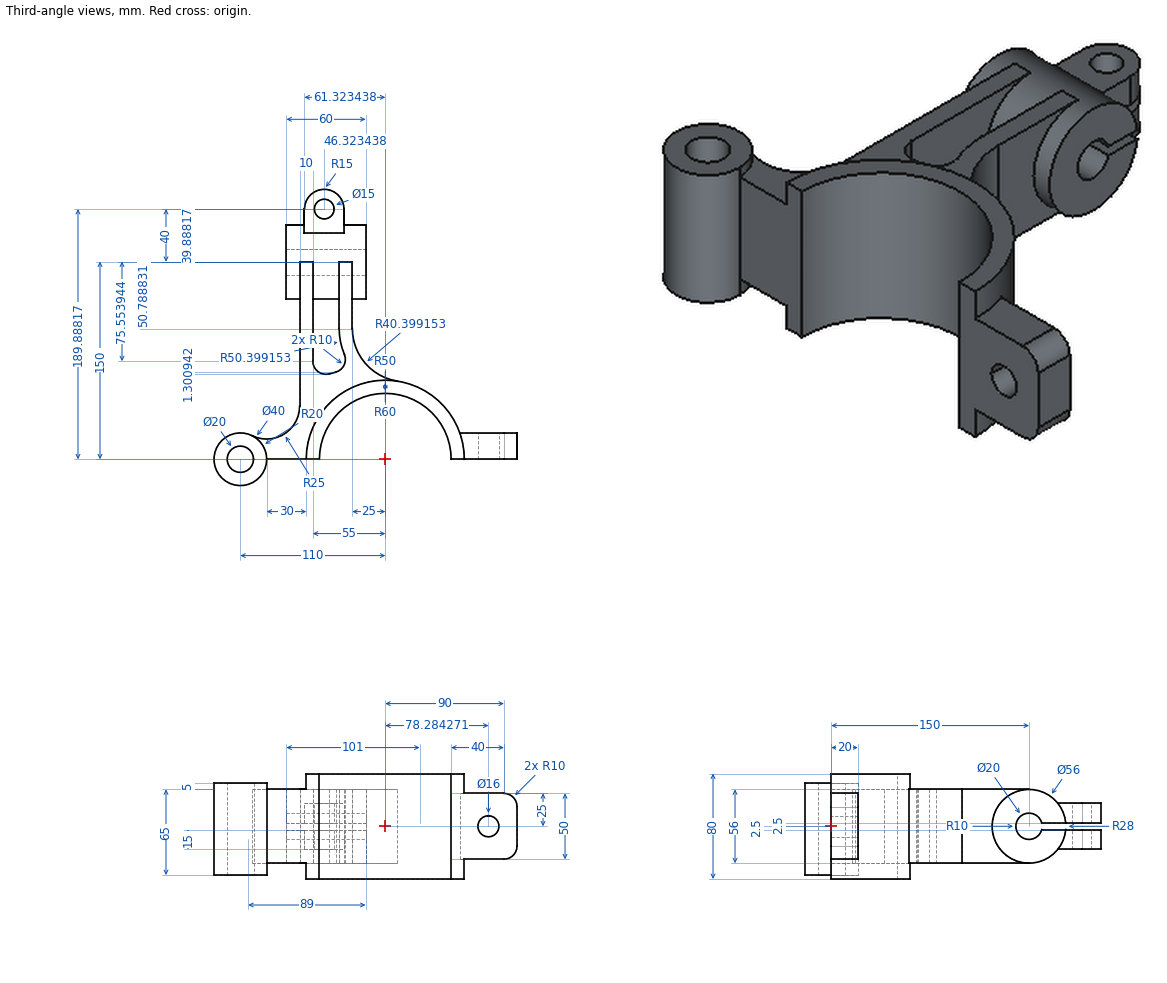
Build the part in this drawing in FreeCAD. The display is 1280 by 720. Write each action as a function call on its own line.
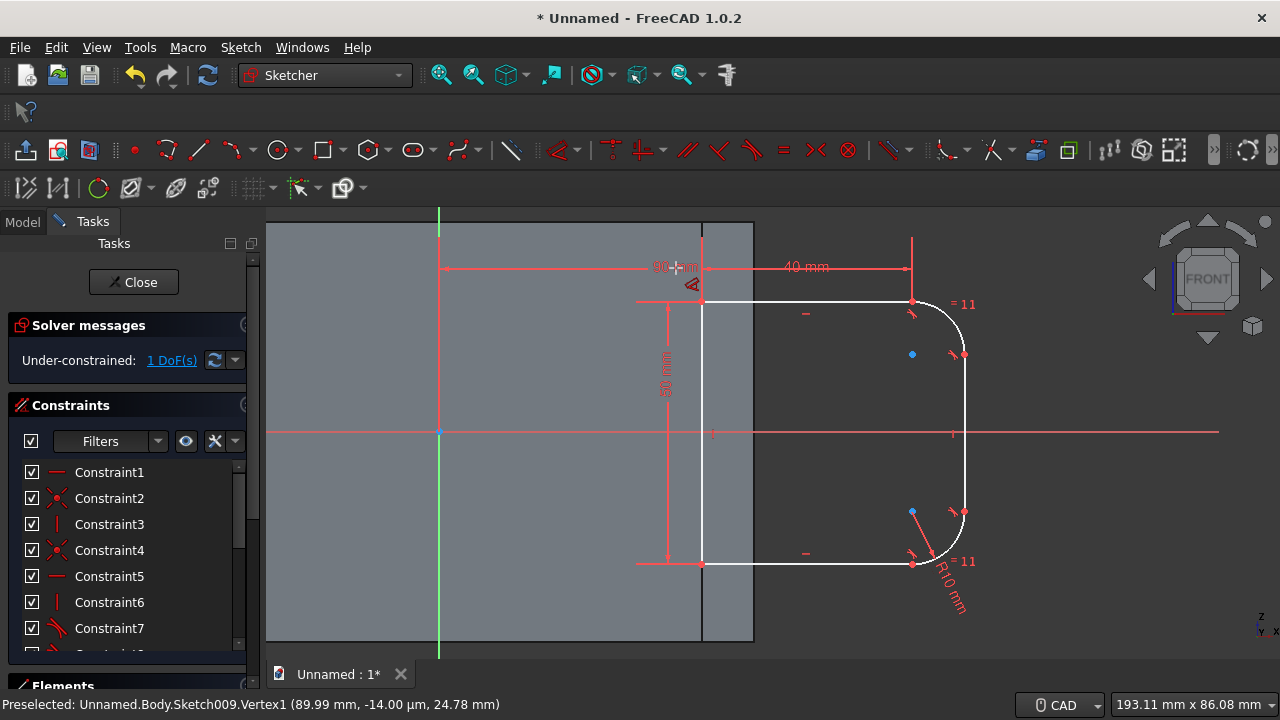
click(912, 302)
click(405, 367)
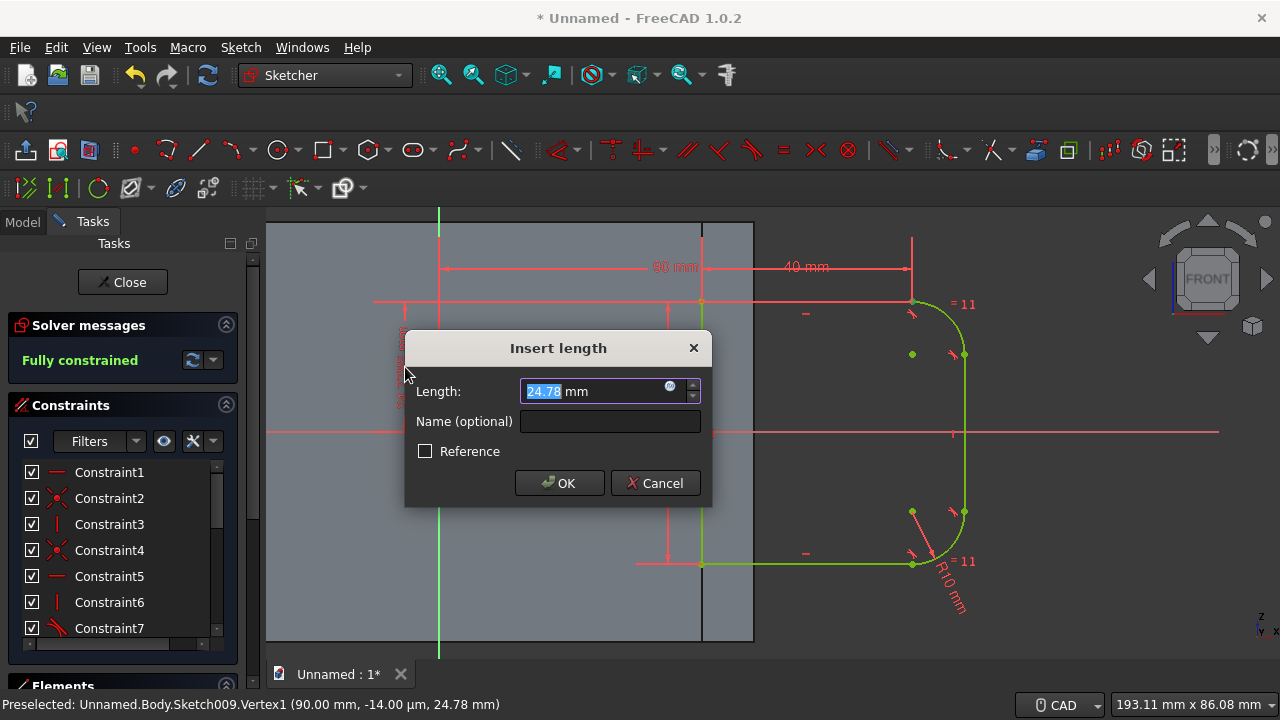
text(25)
key(Return)
key(Escape)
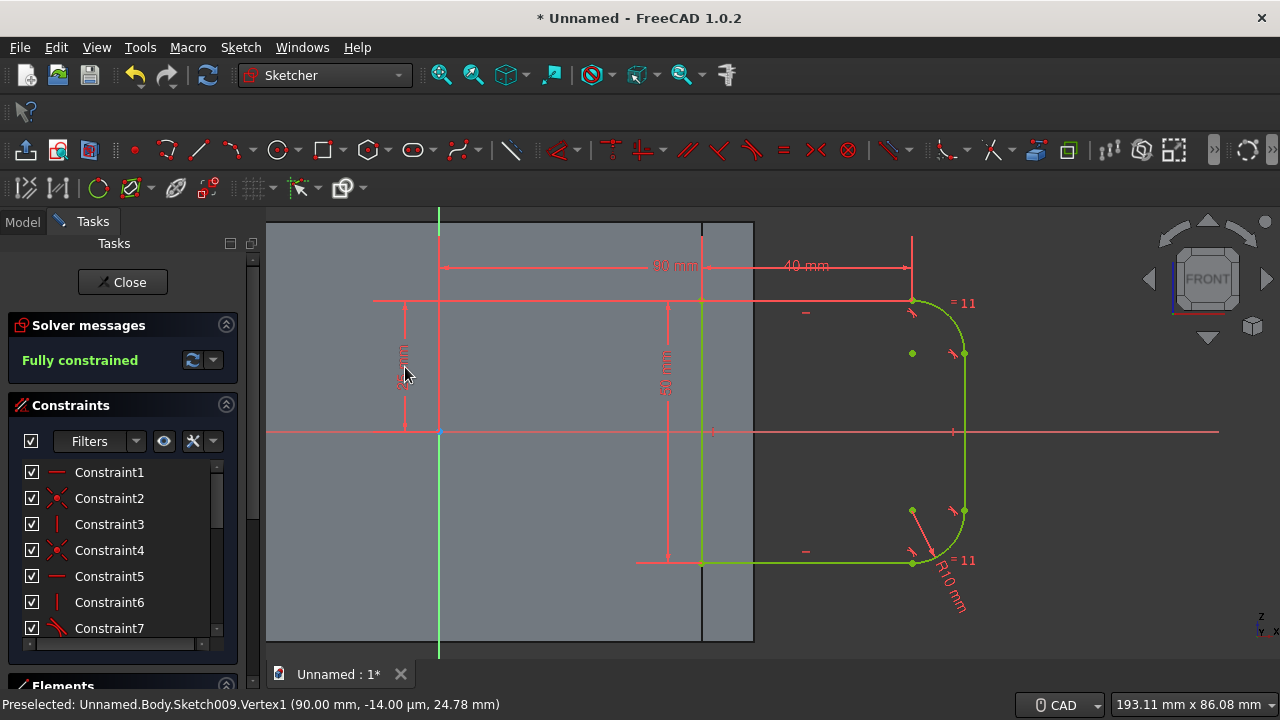
click(123, 282)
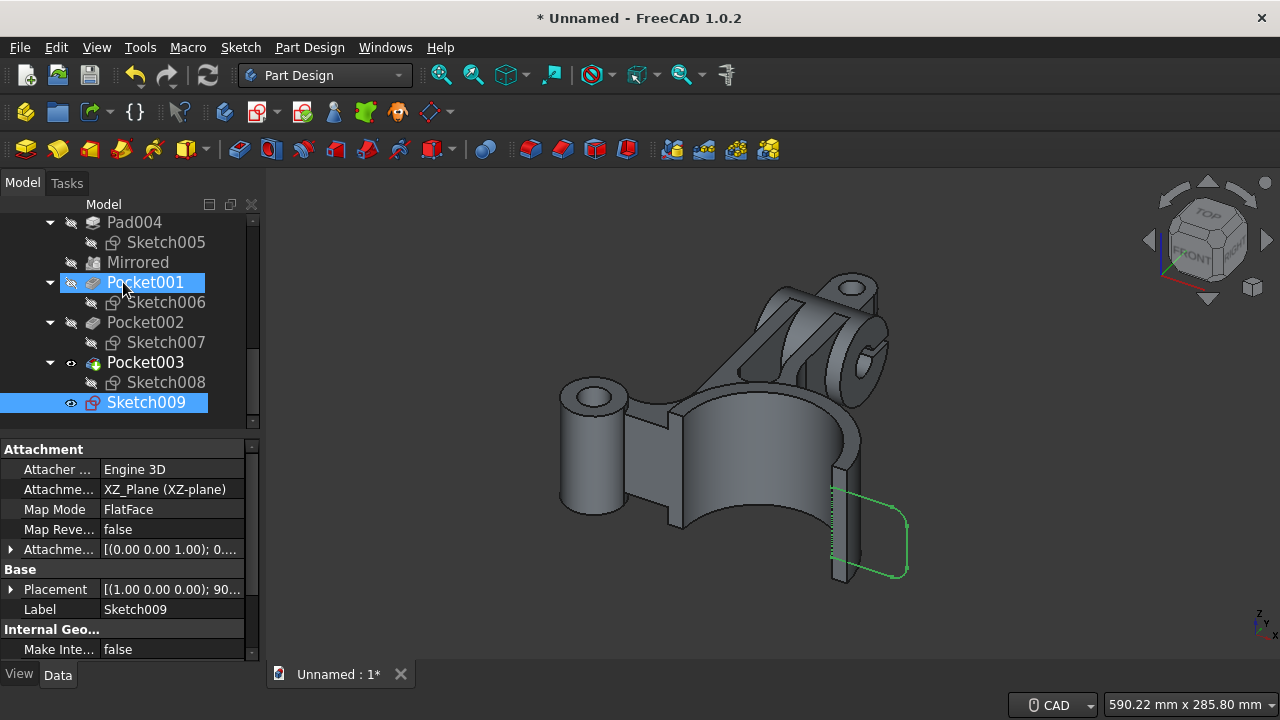
click(26, 150)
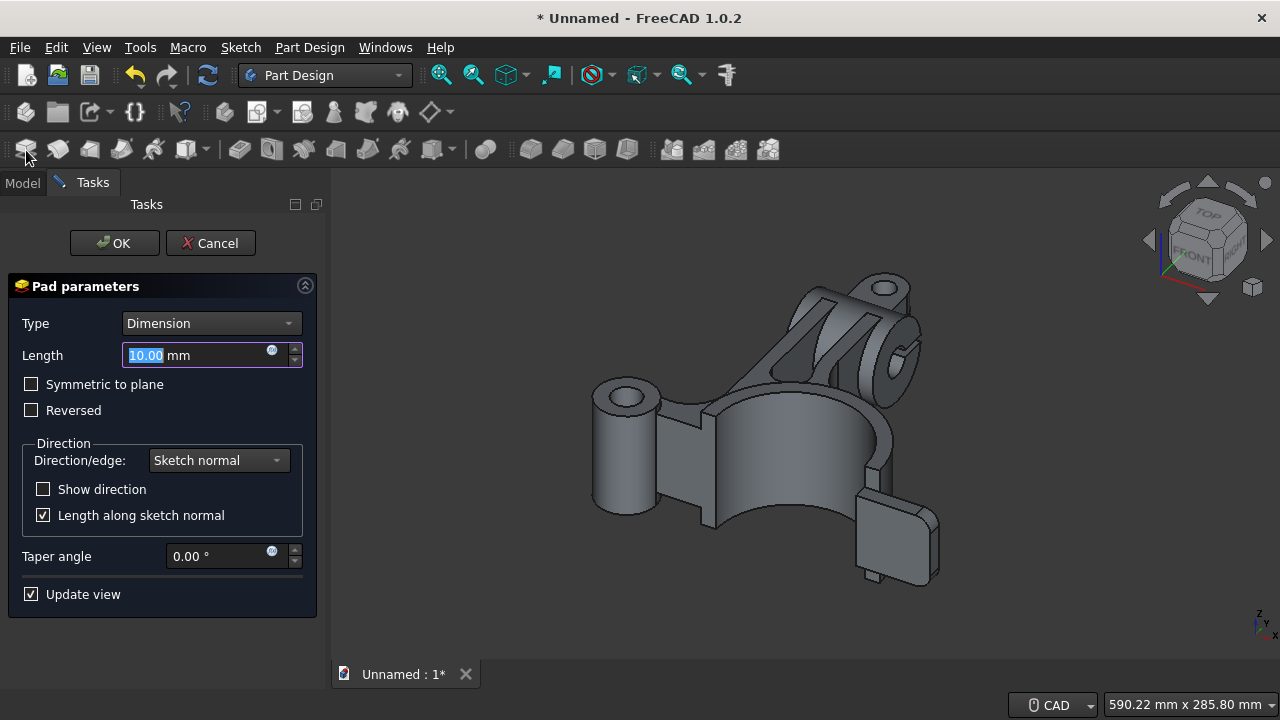
text(20)
key(Tab)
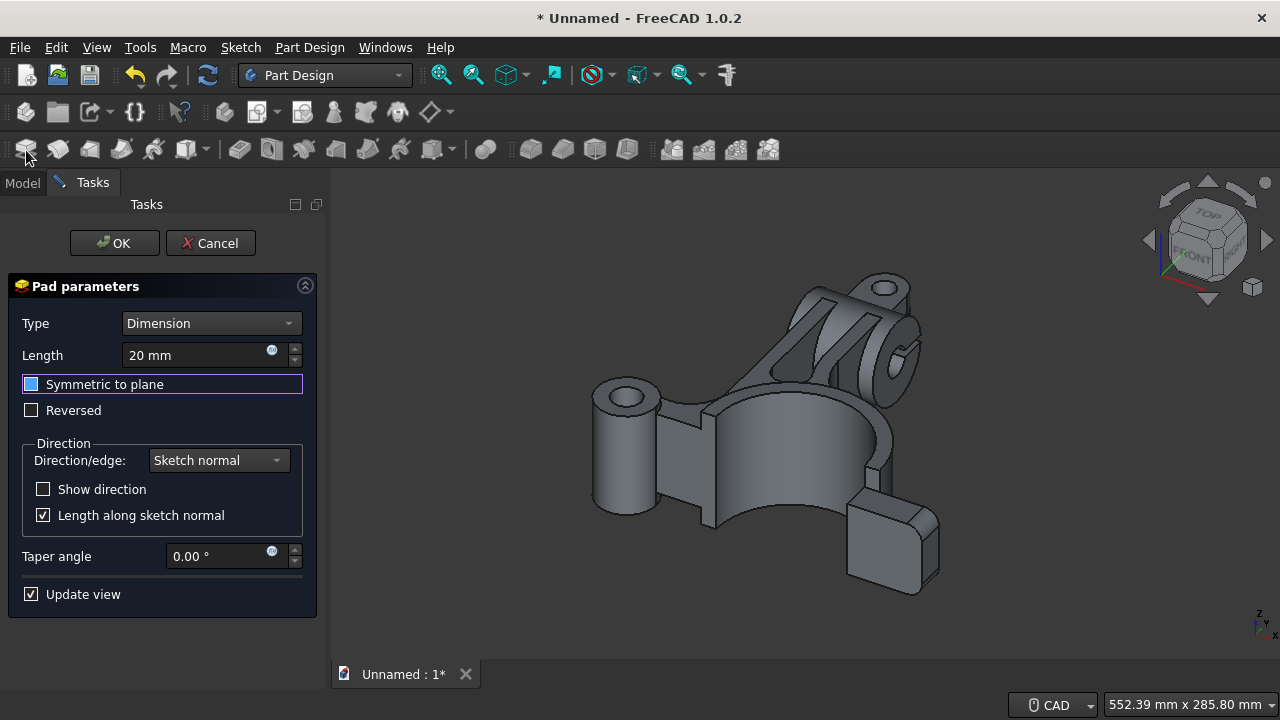
click(30, 410)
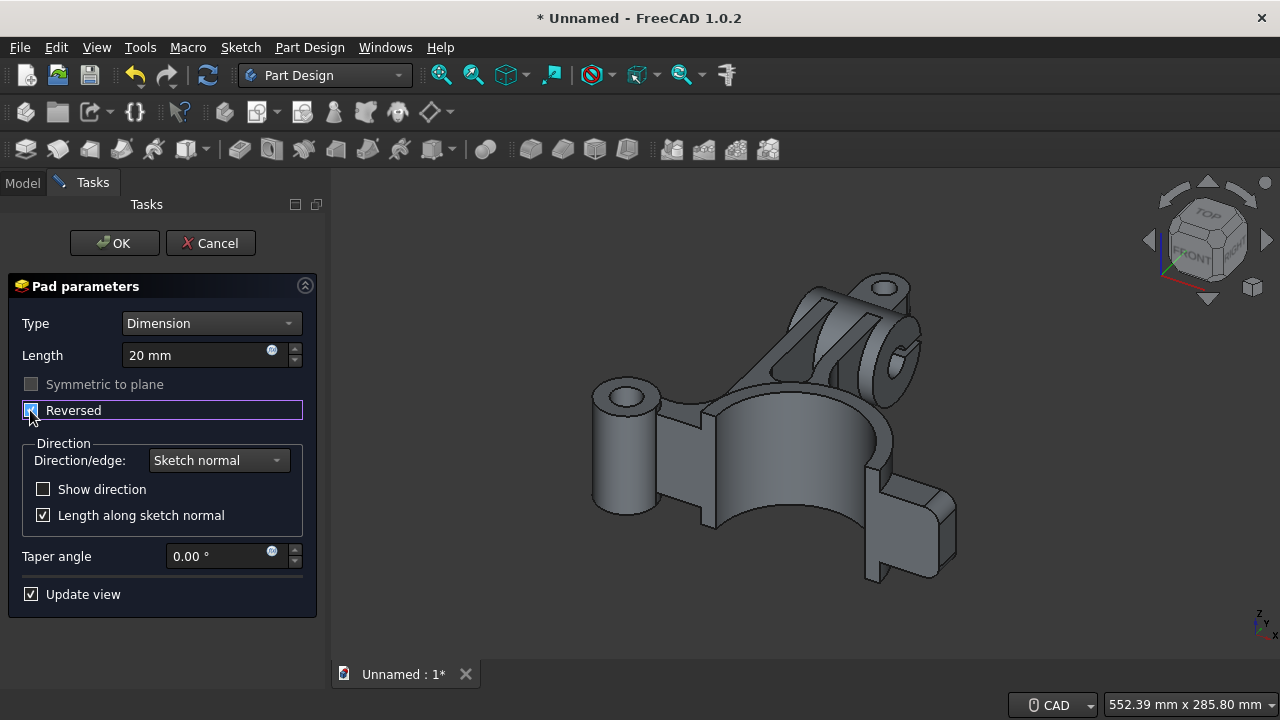
click(115, 243)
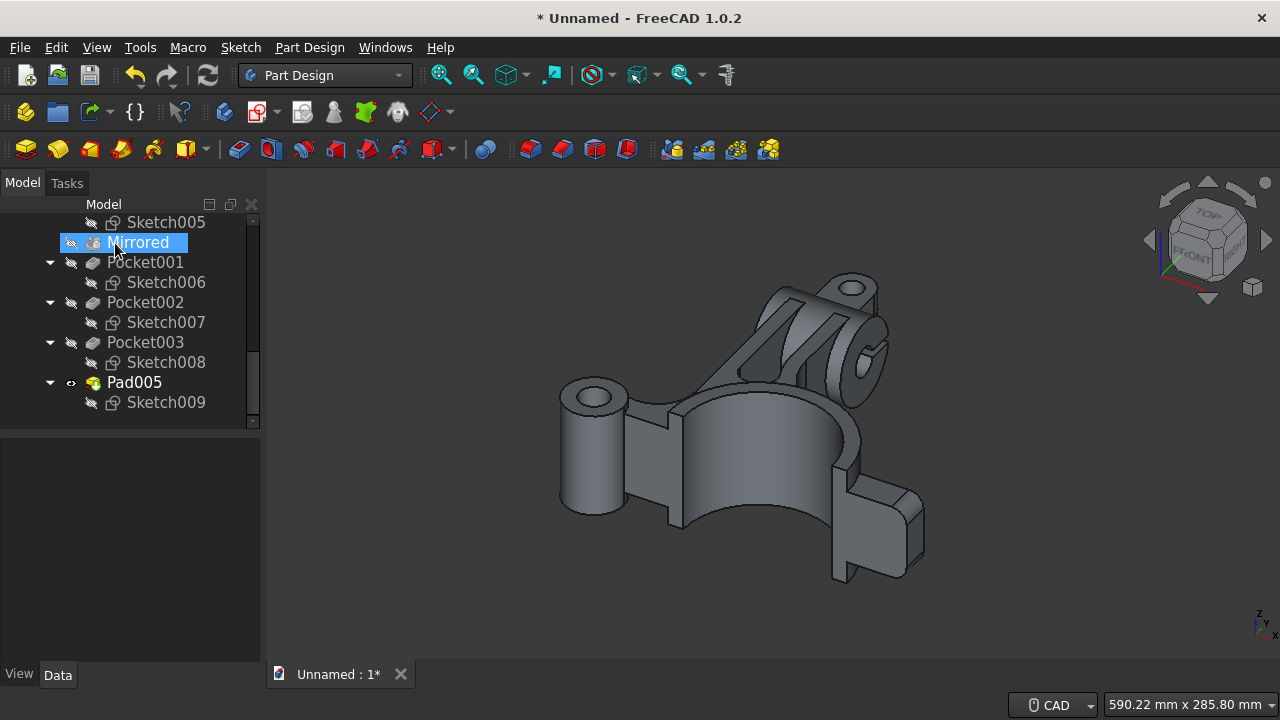
key(4)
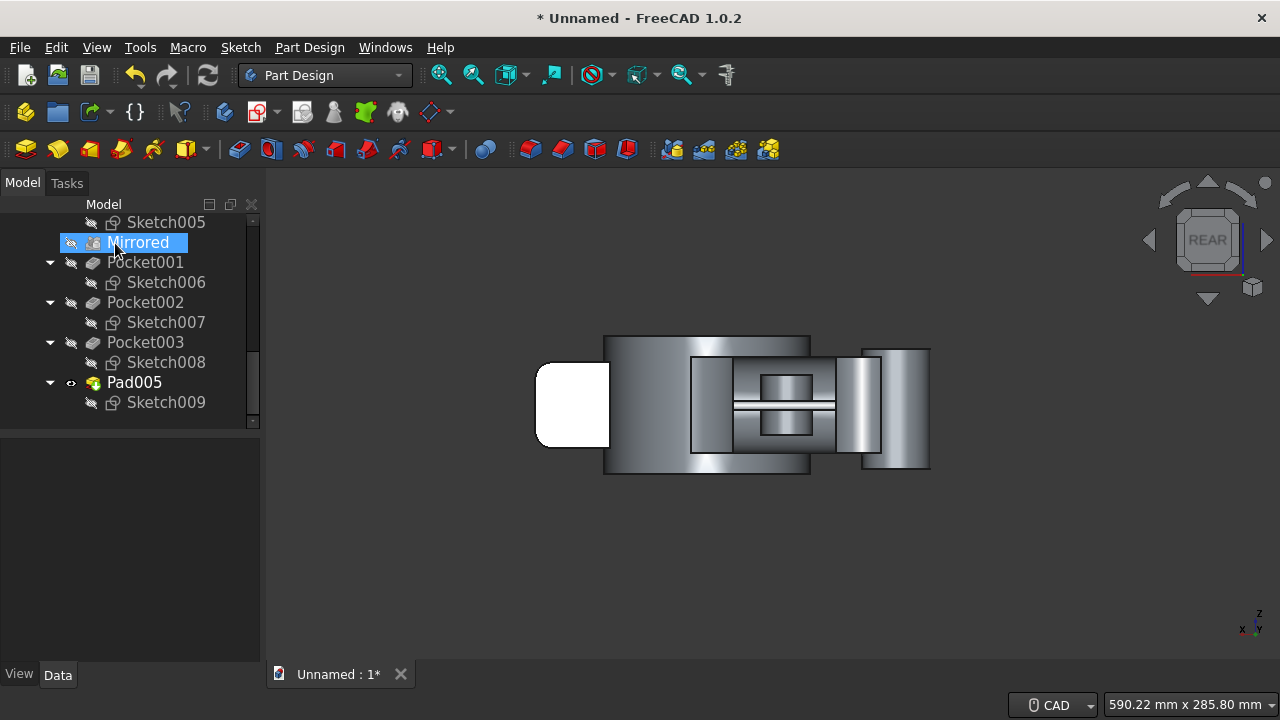
key(v)
key(f)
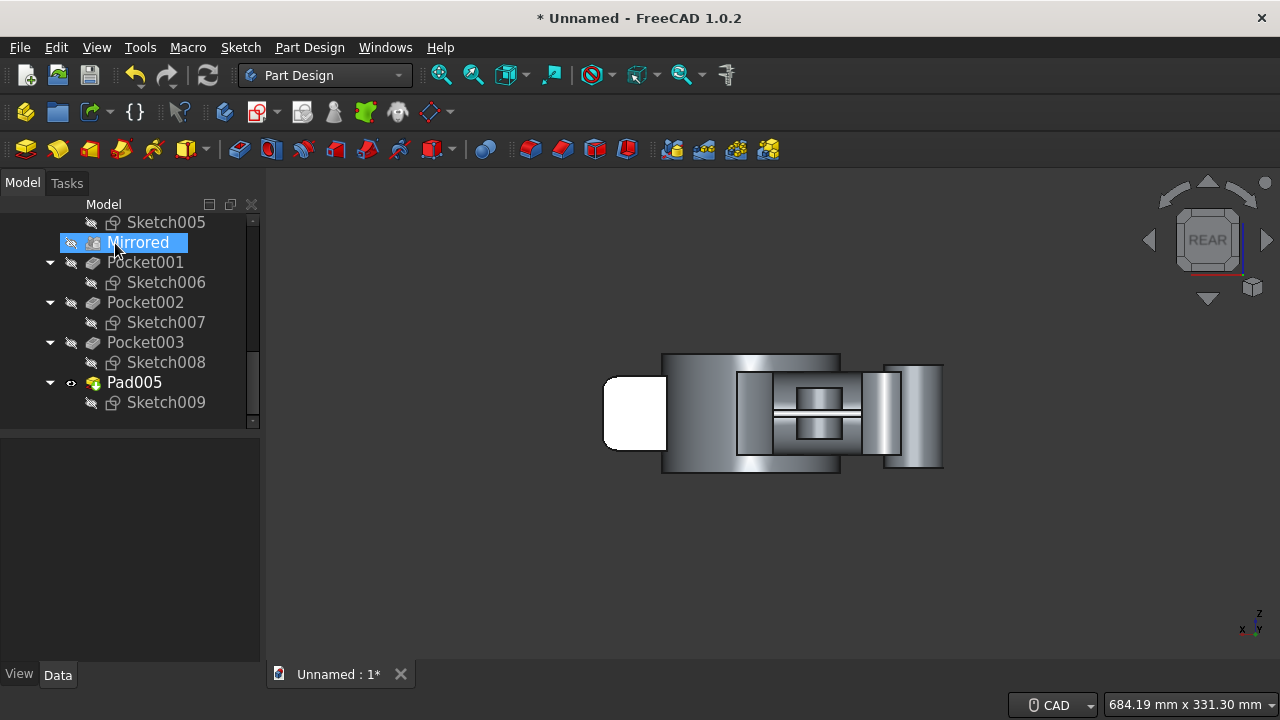
click(635, 413)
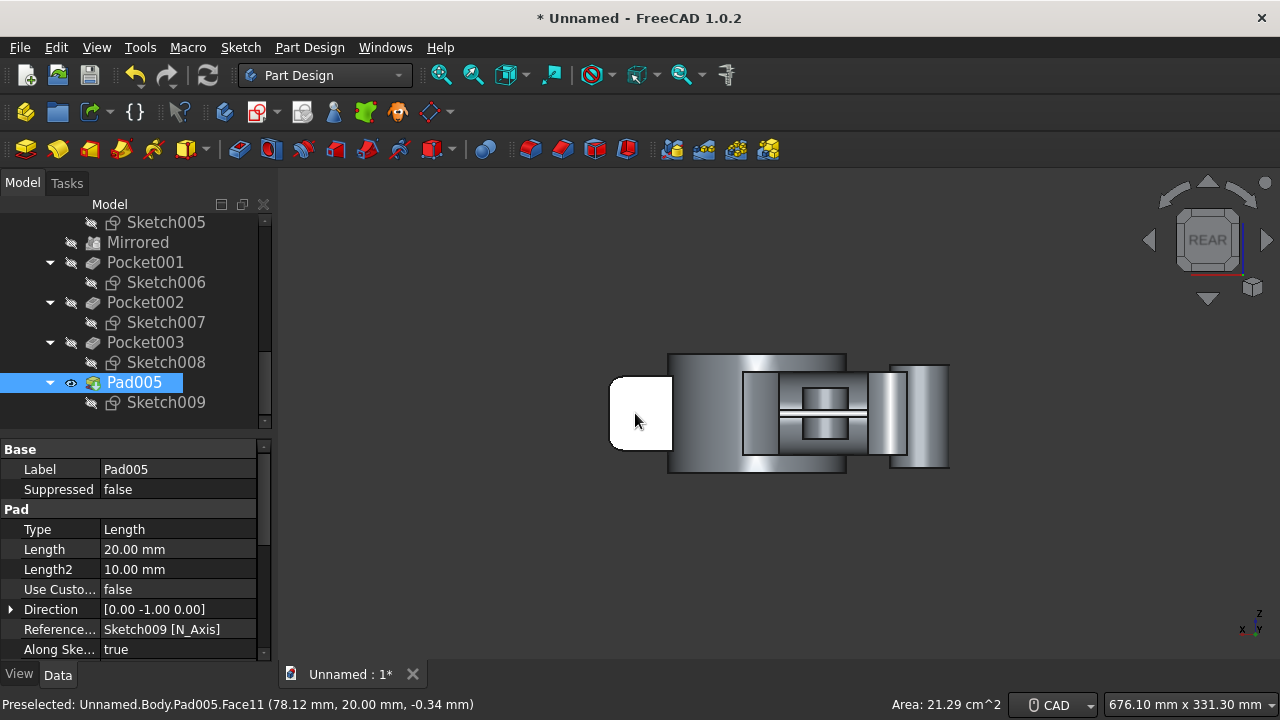
click(258, 112)